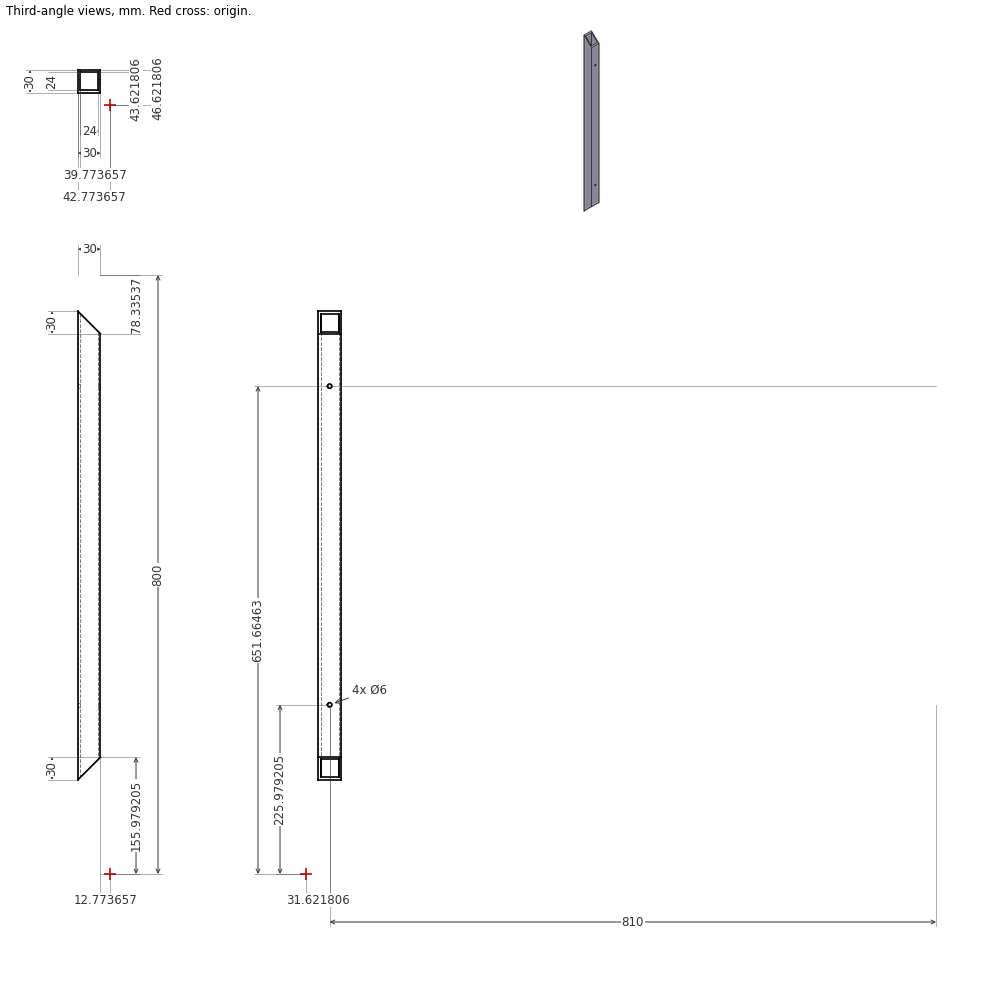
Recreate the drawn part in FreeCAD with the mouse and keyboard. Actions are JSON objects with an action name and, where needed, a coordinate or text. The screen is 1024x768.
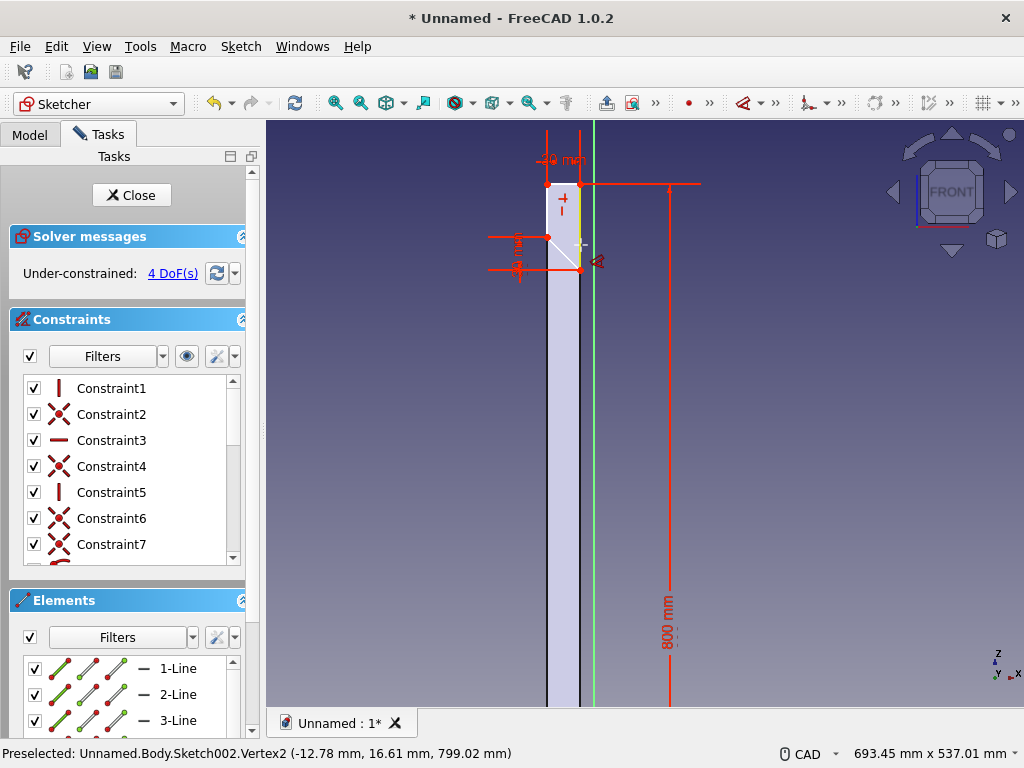
{"action": "left_click", "coordinate": [580, 244]}
{"action": "left_click", "coordinate": [614, 227]}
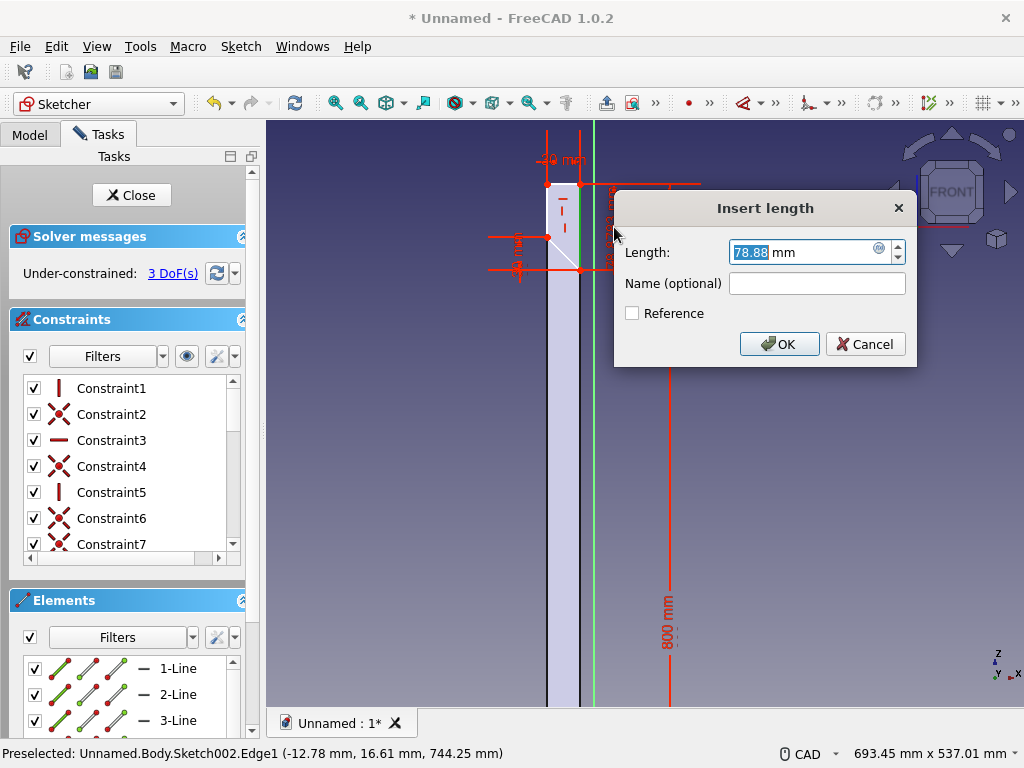
{"action": "type", "text": "78.33537"}
{"action": "key", "text": "Return"}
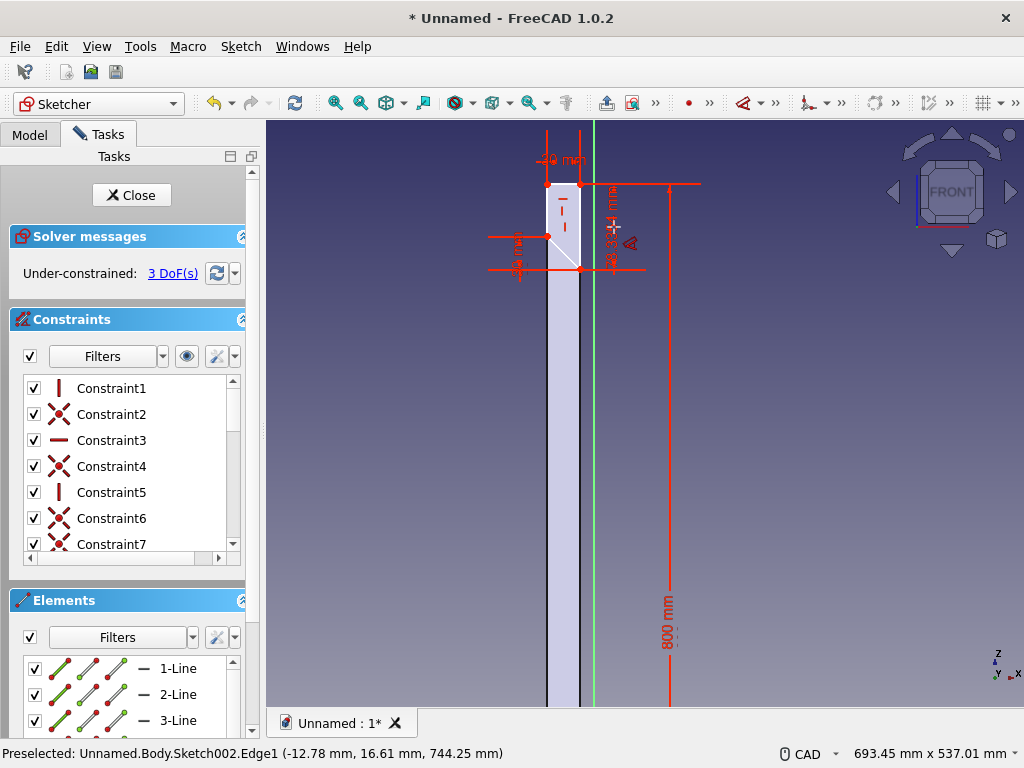
{"action": "scroll", "coordinate": [581, 244], "scroll_direction": "down", "scroll_amount": 4}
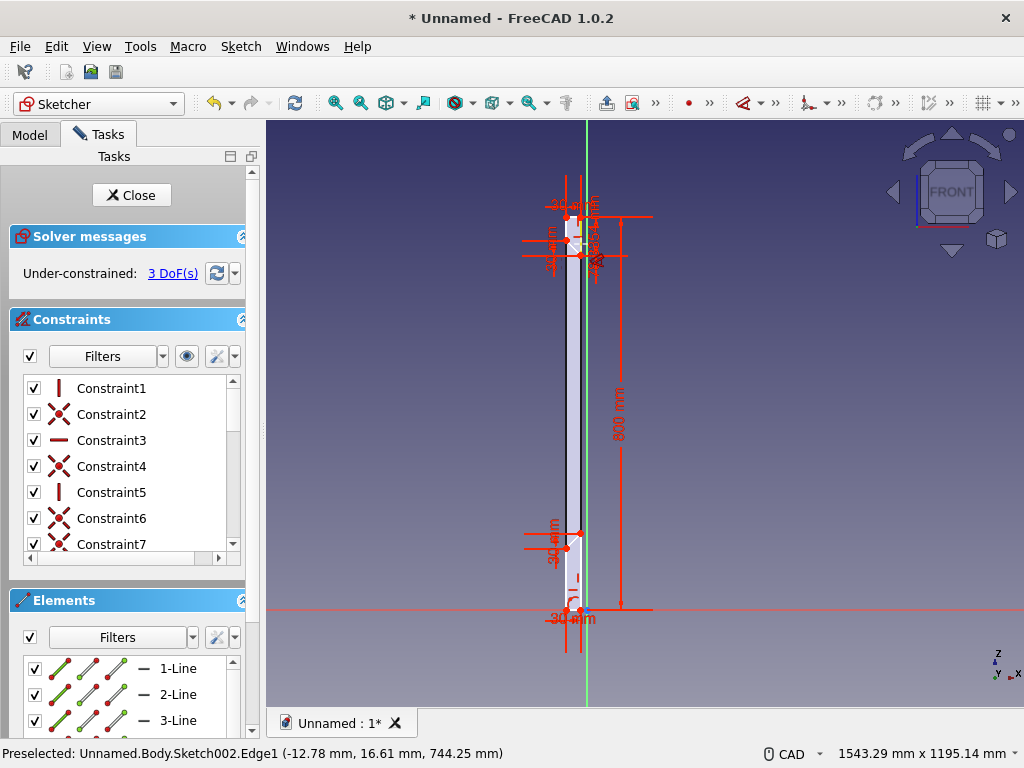
{"action": "scroll", "coordinate": [581, 587], "scroll_direction": "up", "scroll_amount": 4}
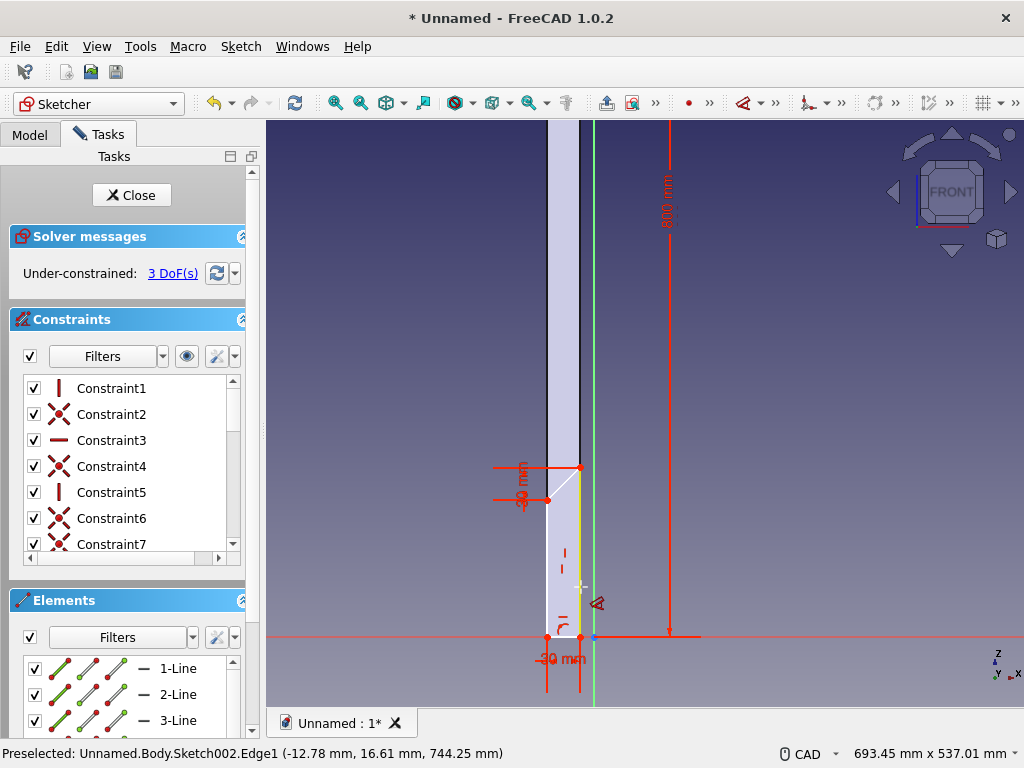
{"action": "left_click", "coordinate": [580, 586]}
{"action": "left_click", "coordinate": [614, 553]}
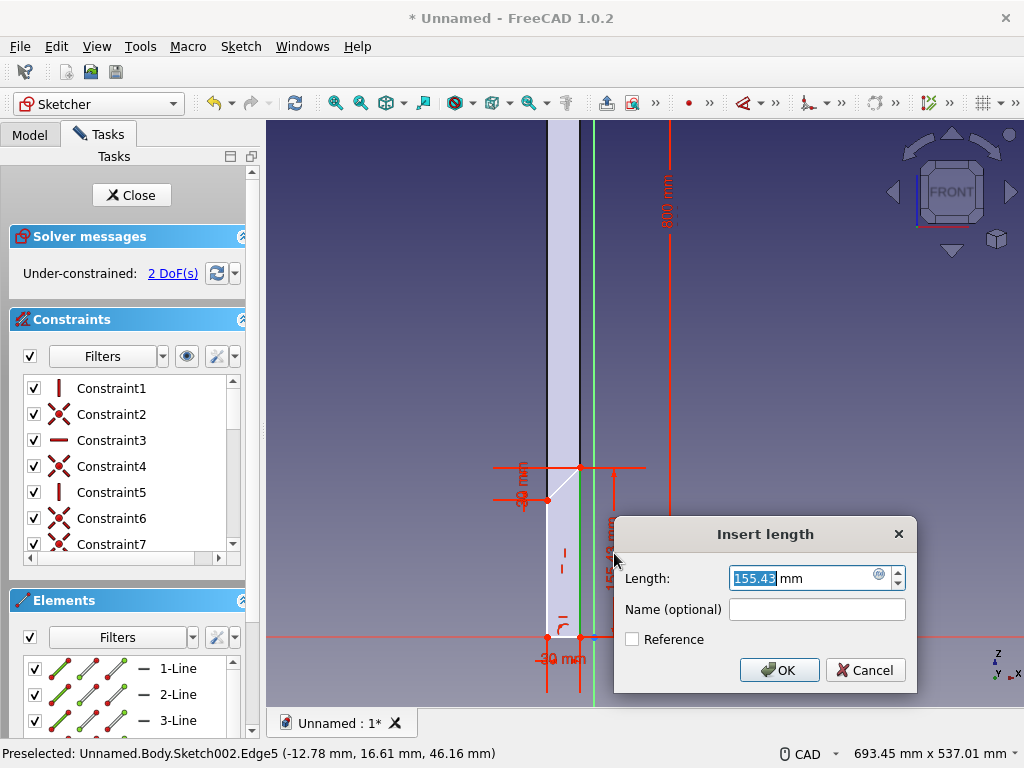
{"action": "type", "text": "155.979205"}
{"action": "key", "text": "Return"}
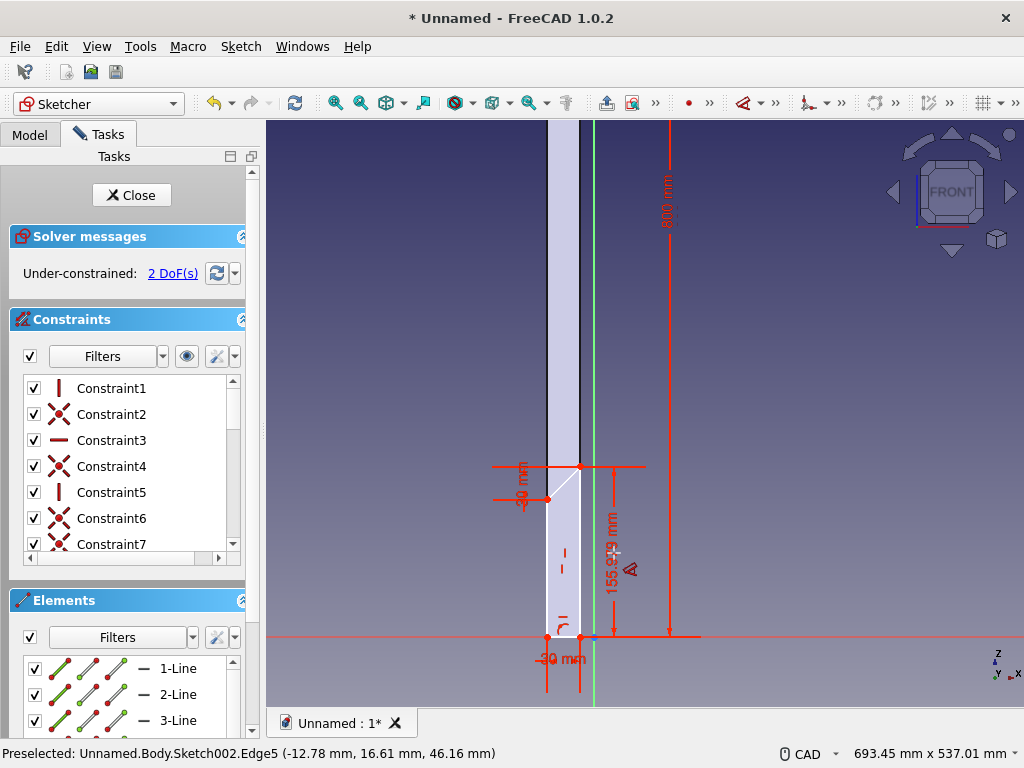
{"action": "scroll", "coordinate": [581, 588], "scroll_direction": "down", "scroll_amount": 4}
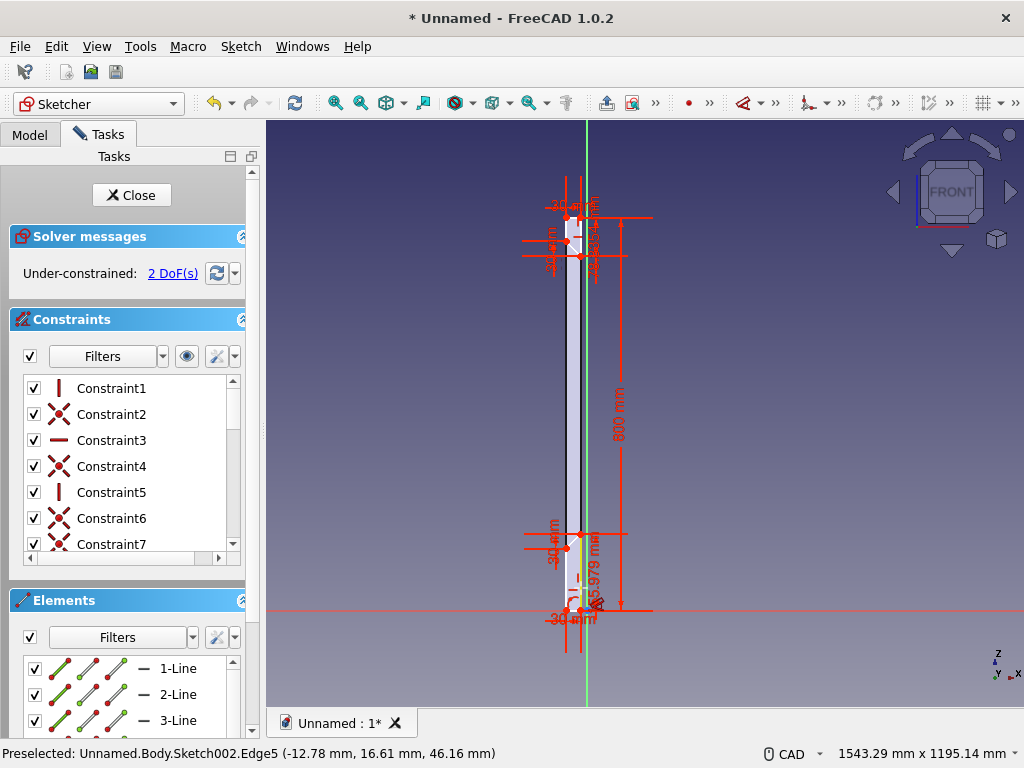
{"action": "scroll", "coordinate": [581, 256], "scroll_direction": "up", "scroll_amount": 10}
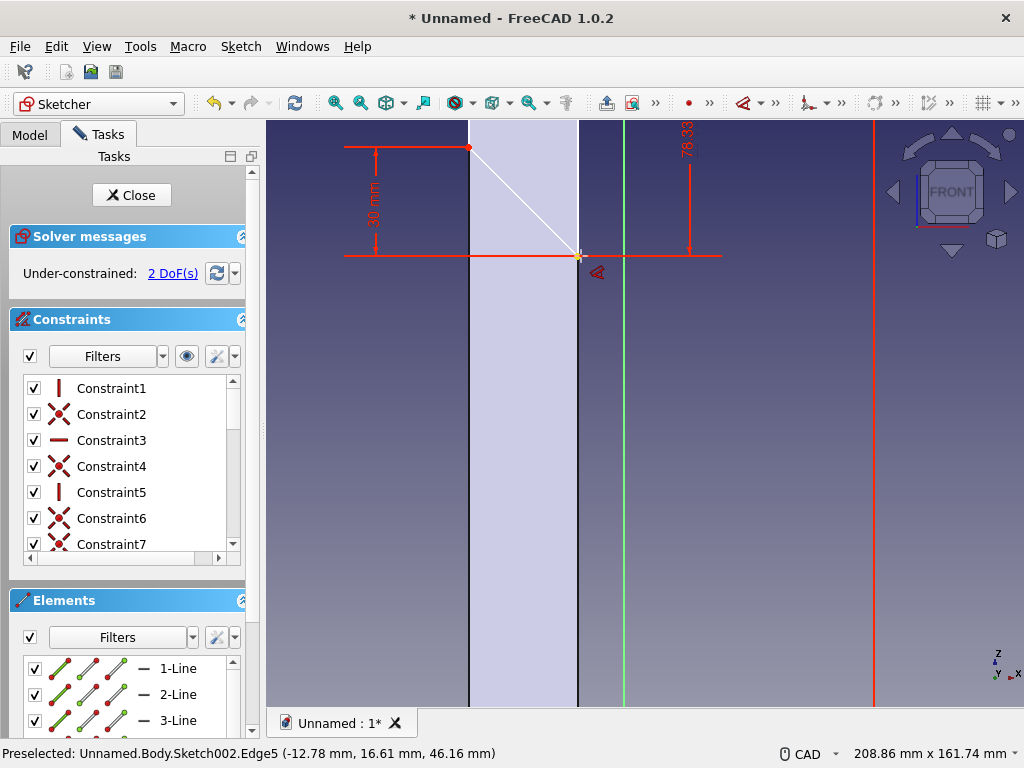
{"action": "left_click", "coordinate": [578, 256]}
{"action": "left_click", "coordinate": [601, 222]}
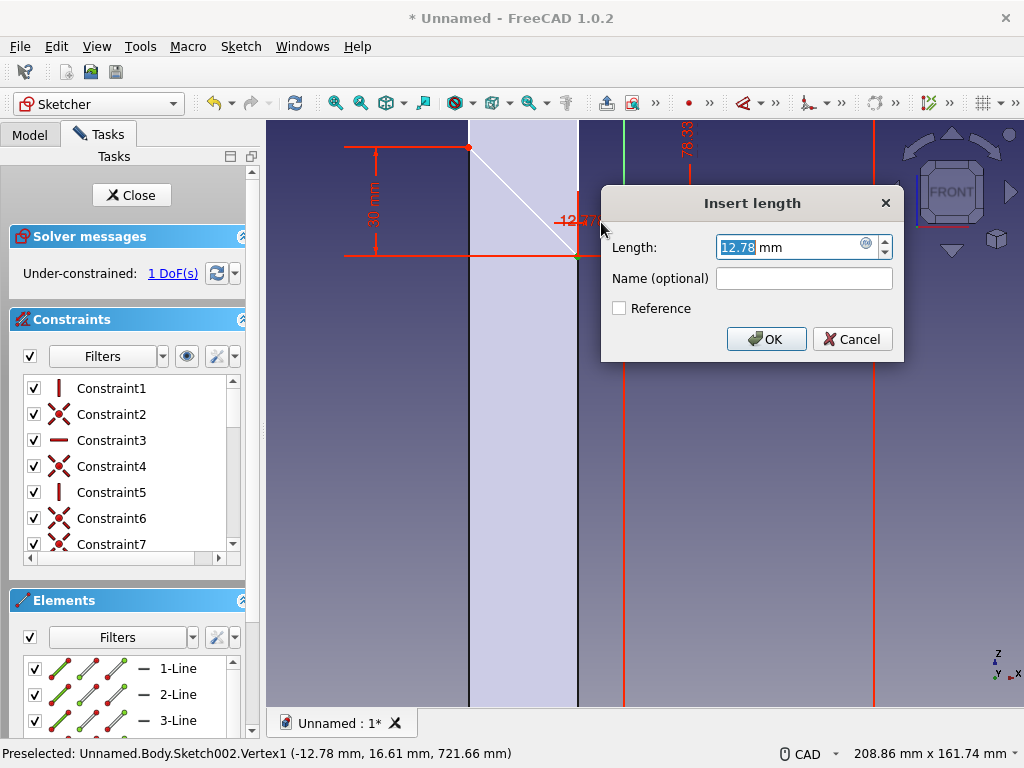
{"action": "type", "text": "12.773657"}
{"action": "key", "text": "Return"}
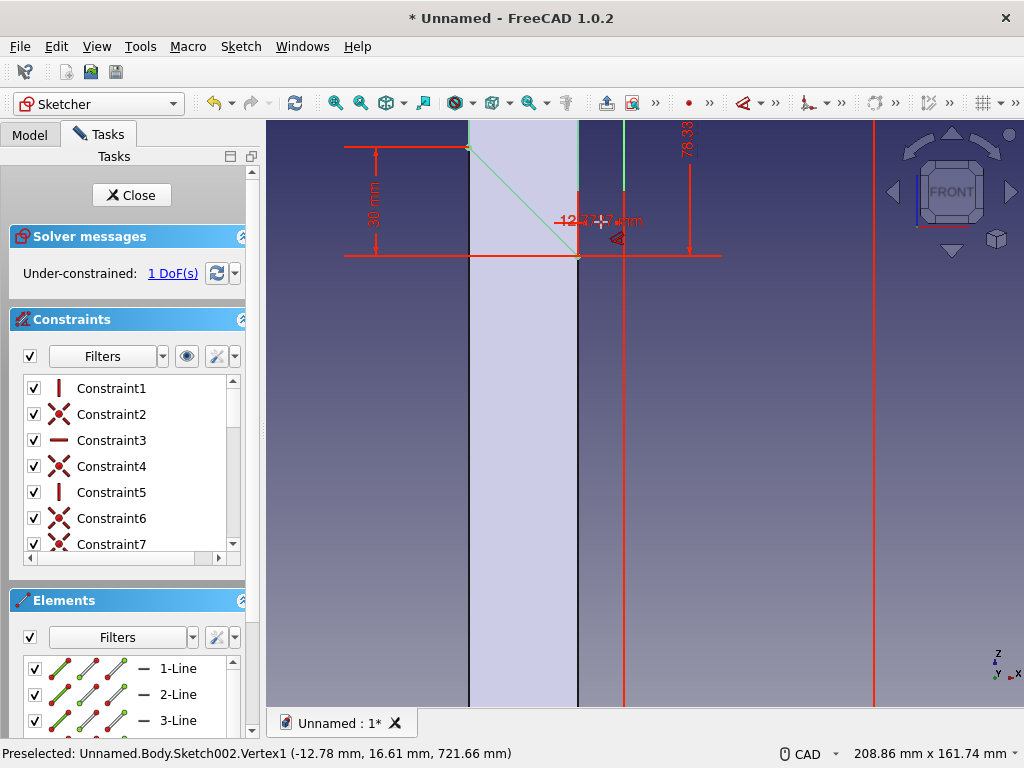
{"action": "scroll", "coordinate": [581, 255], "scroll_direction": "down", "scroll_amount": 10}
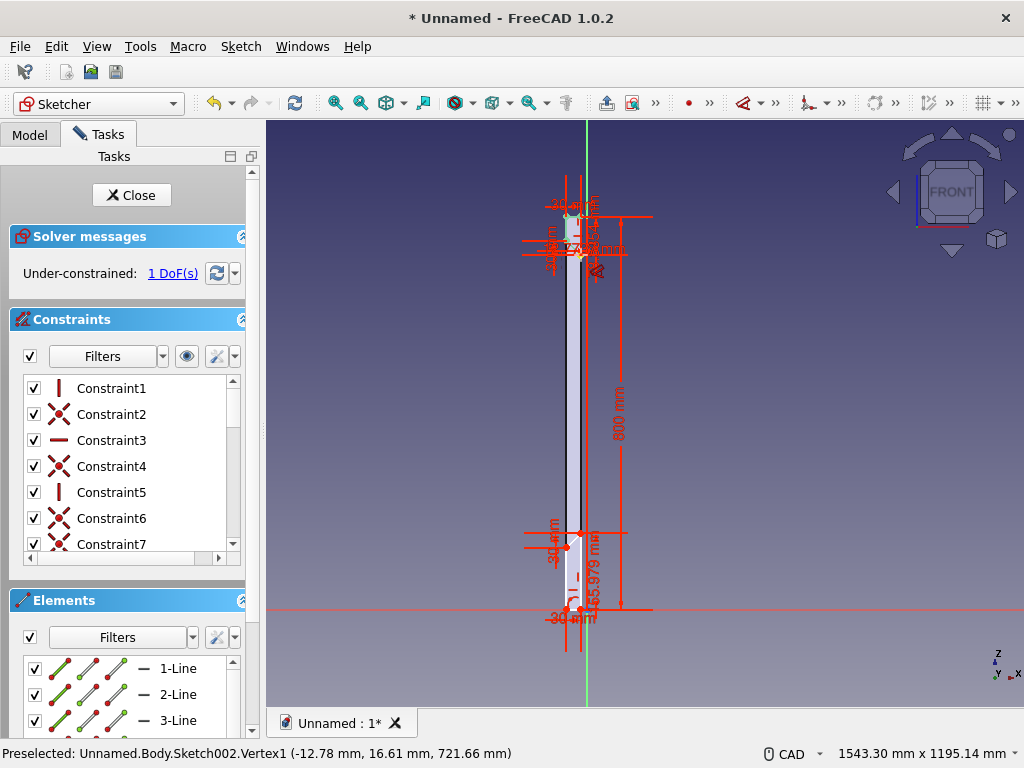
{"action": "scroll", "coordinate": [581, 610], "scroll_direction": "up", "scroll_amount": 10}